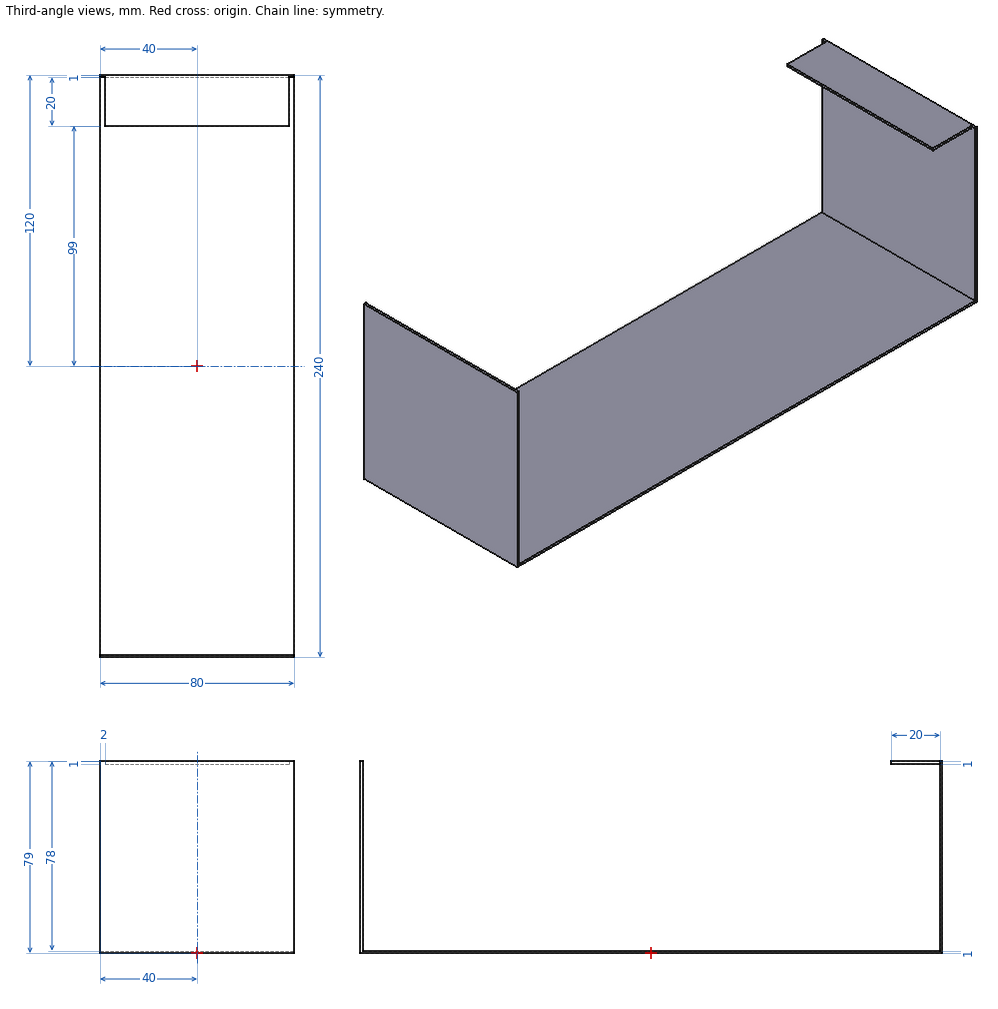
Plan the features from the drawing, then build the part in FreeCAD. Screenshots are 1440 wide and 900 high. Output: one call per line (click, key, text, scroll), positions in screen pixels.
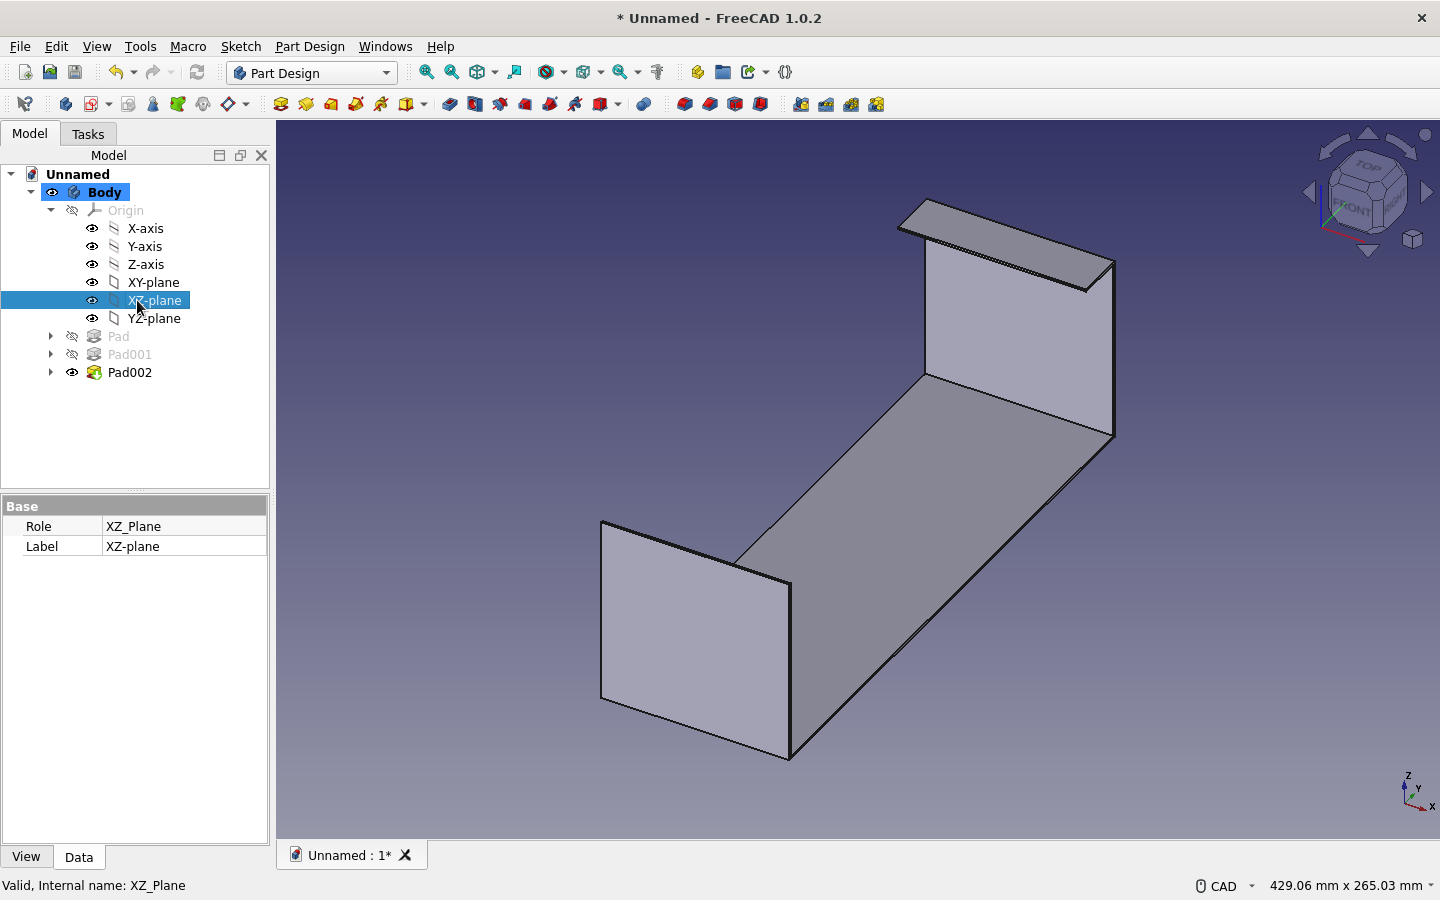
click(228, 104)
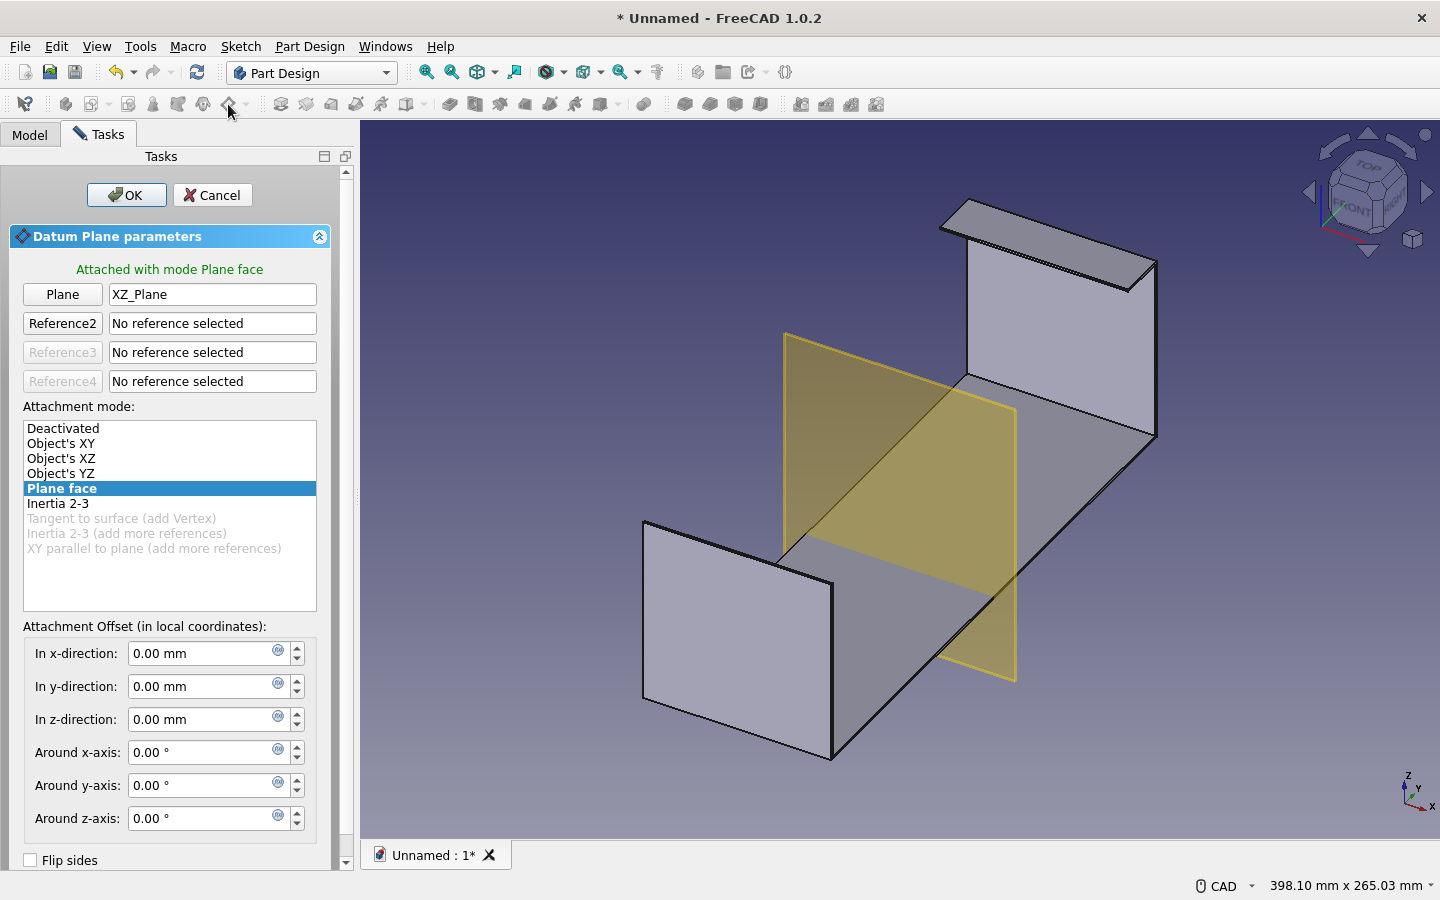
triple_click(210, 720)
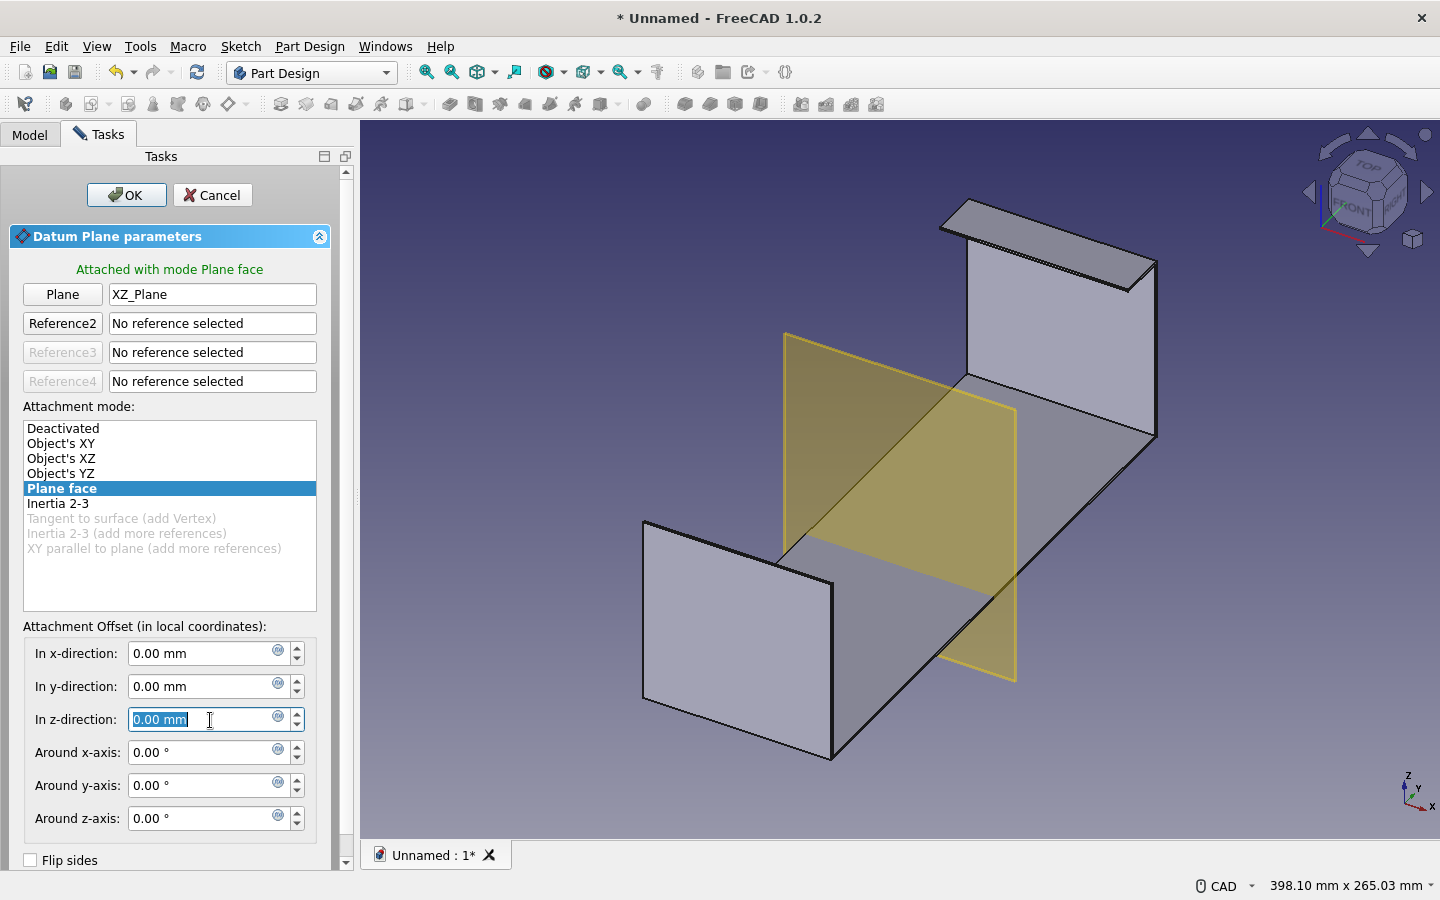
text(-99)
key(Tab)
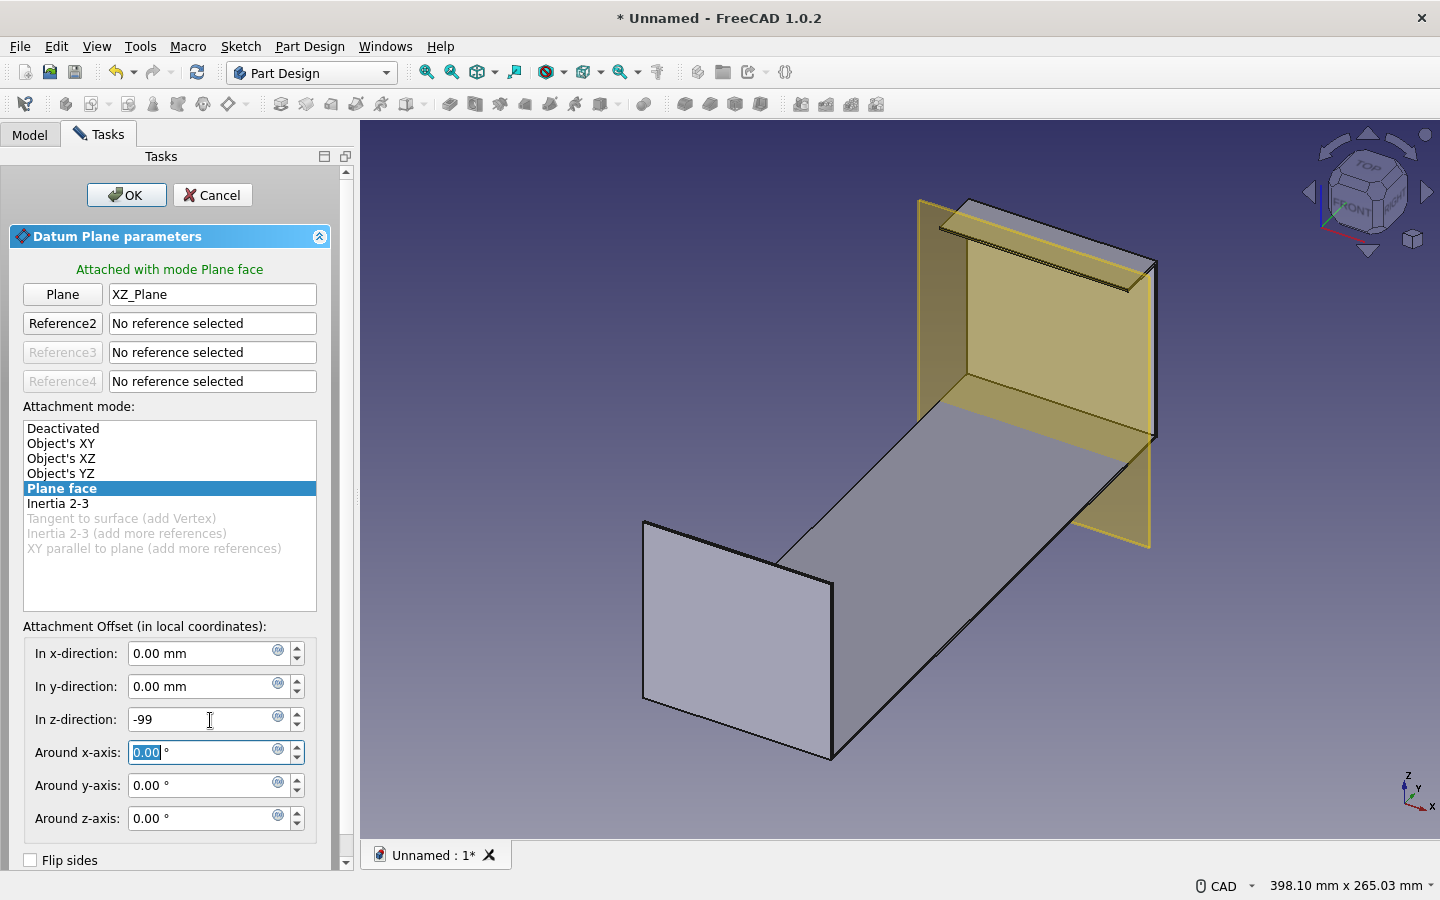
click(127, 195)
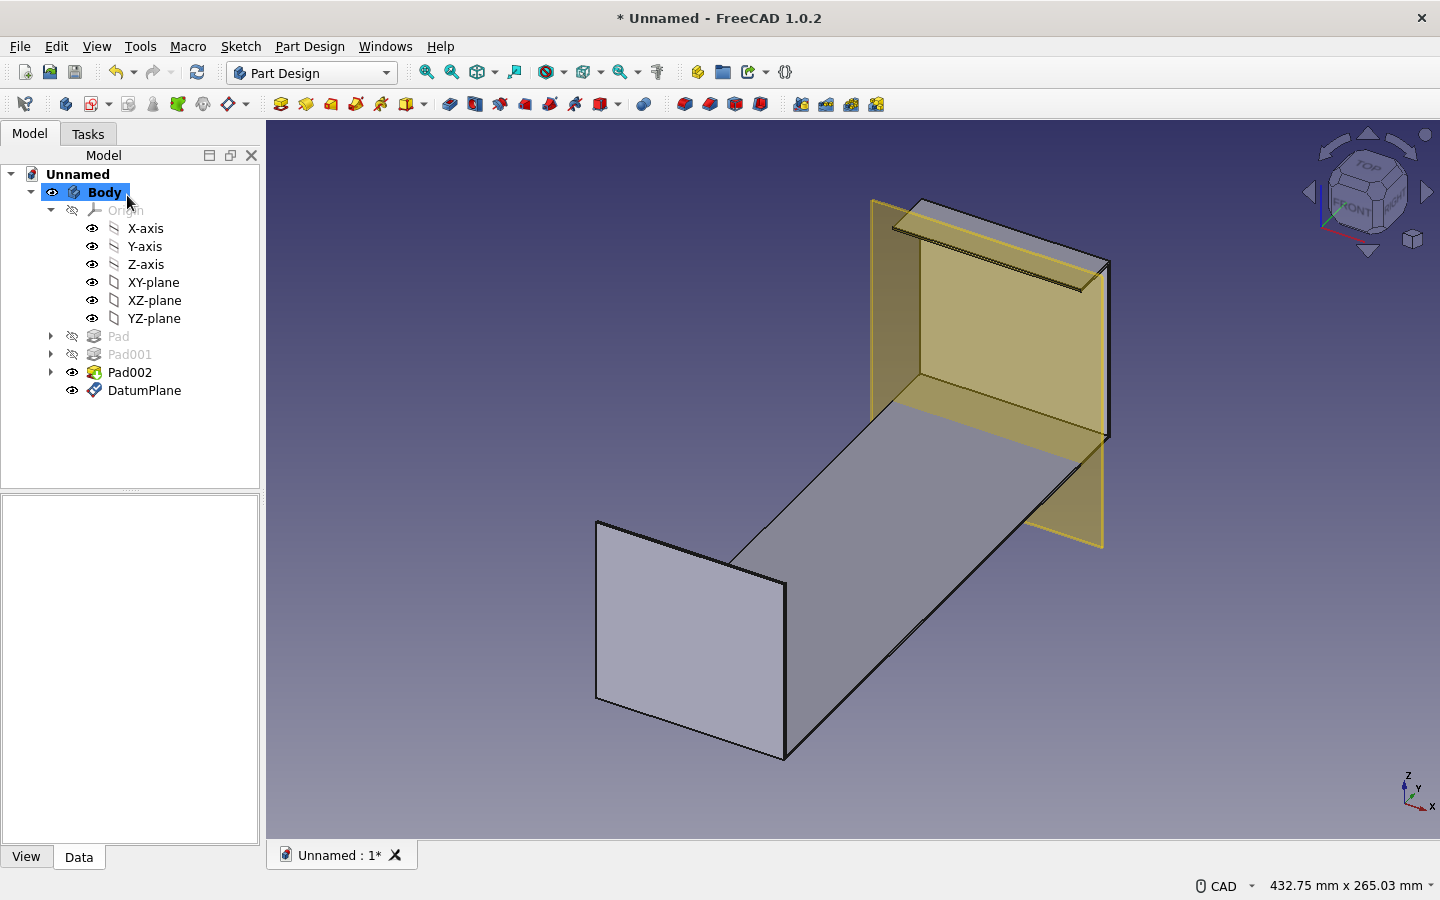
click(117, 390)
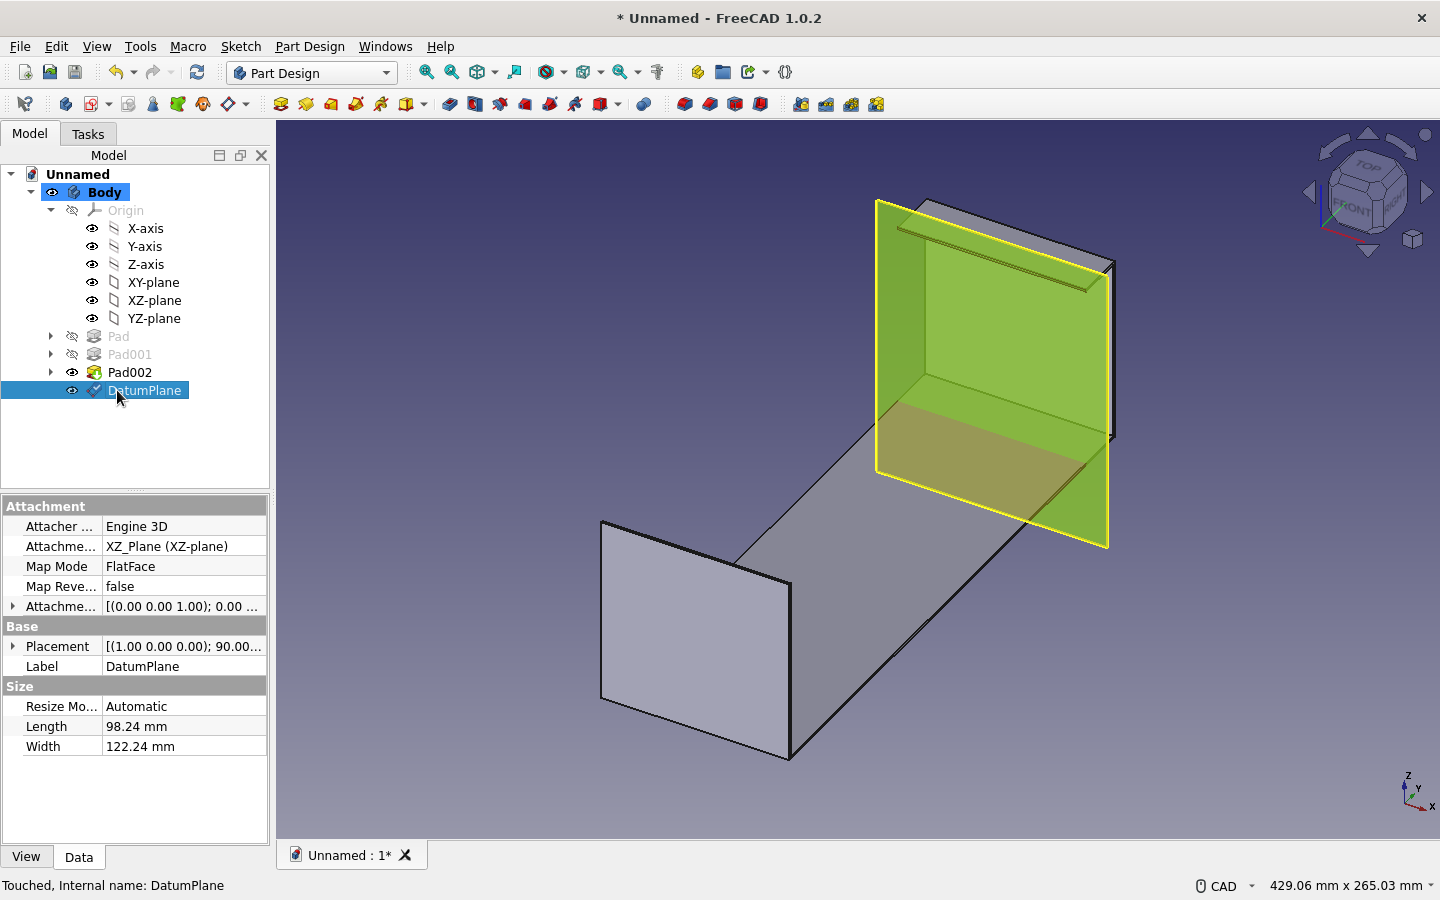
click(90, 104)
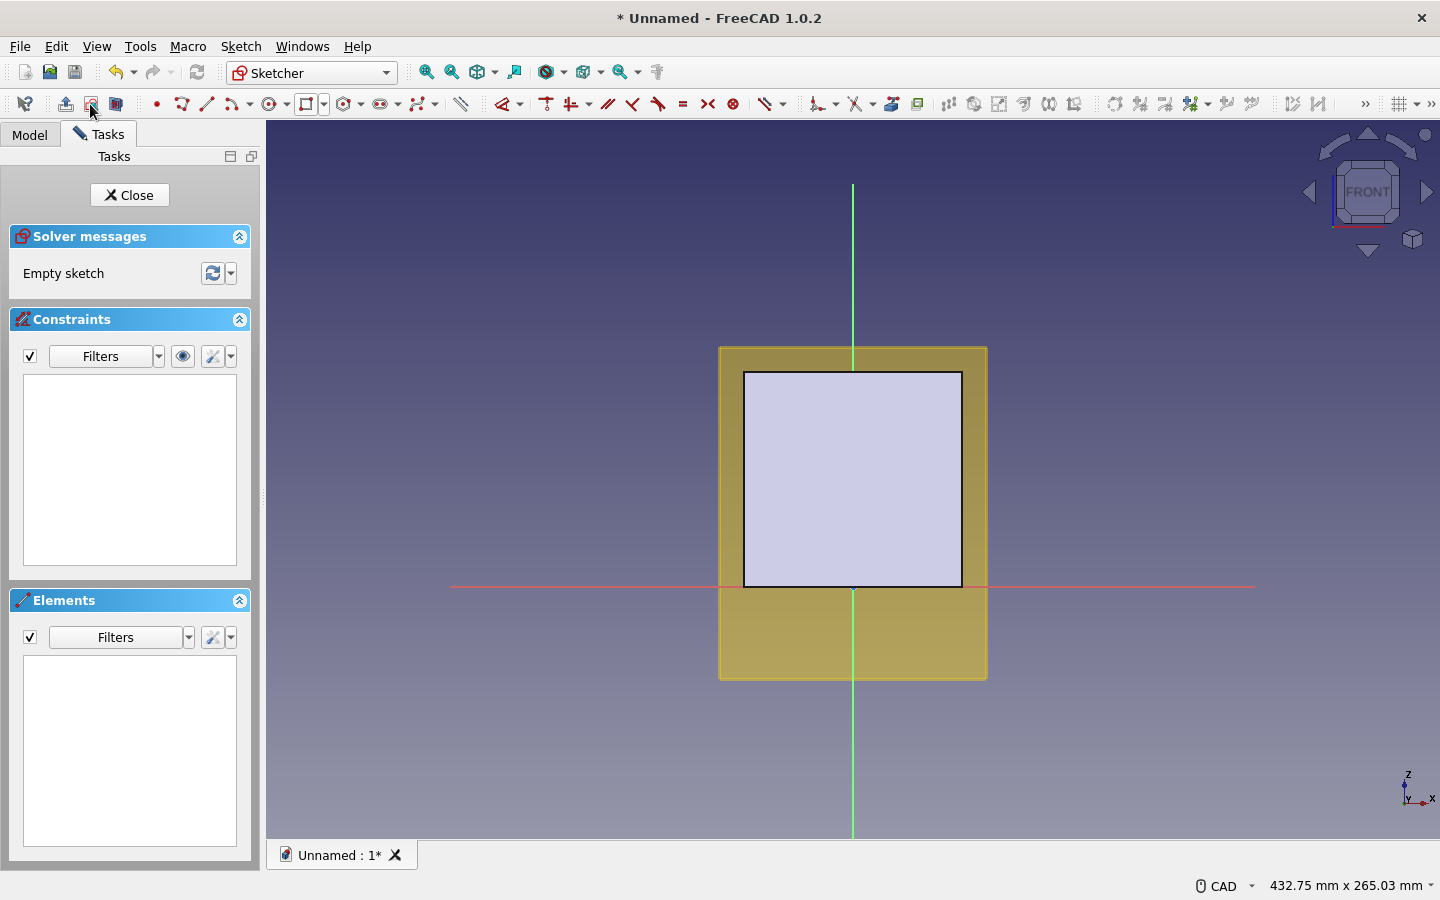
key(q)
key(s)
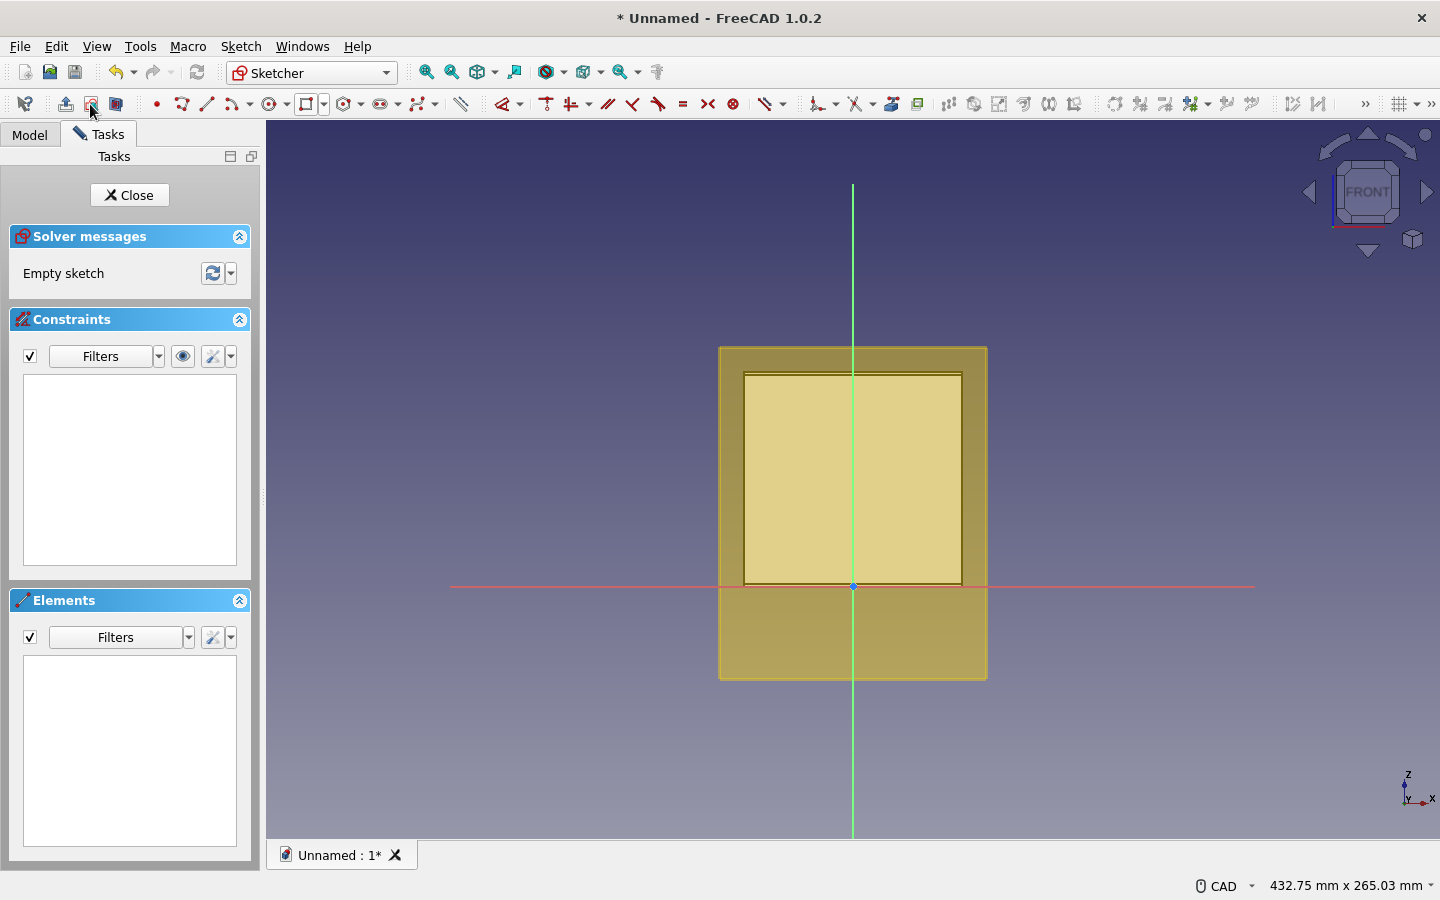
scroll(909, 480, up, 4)